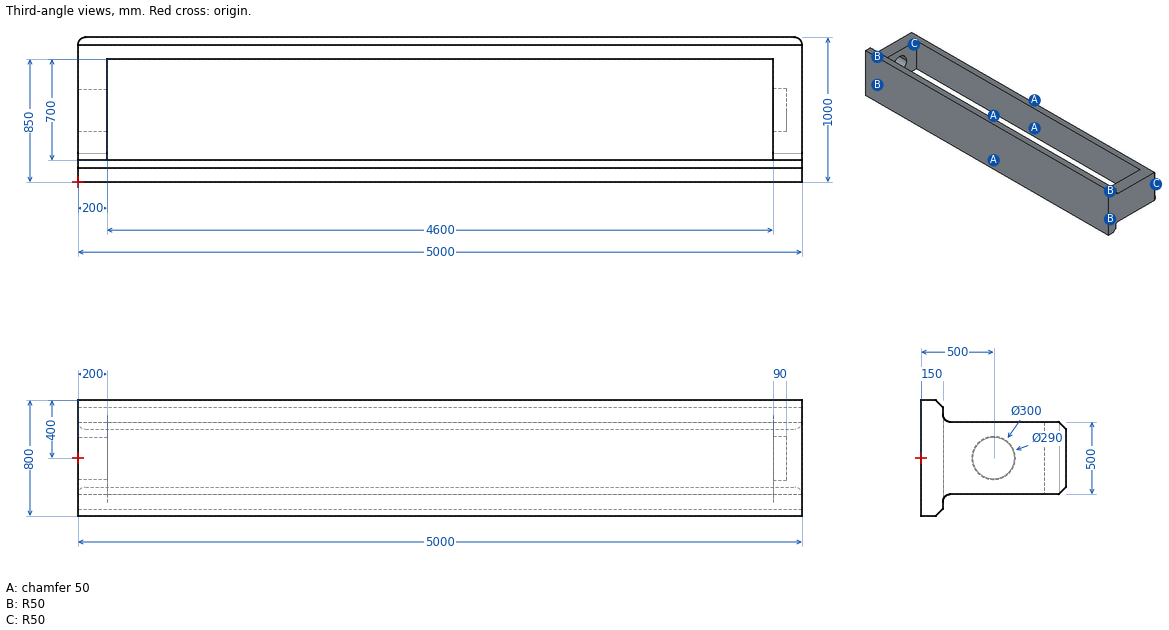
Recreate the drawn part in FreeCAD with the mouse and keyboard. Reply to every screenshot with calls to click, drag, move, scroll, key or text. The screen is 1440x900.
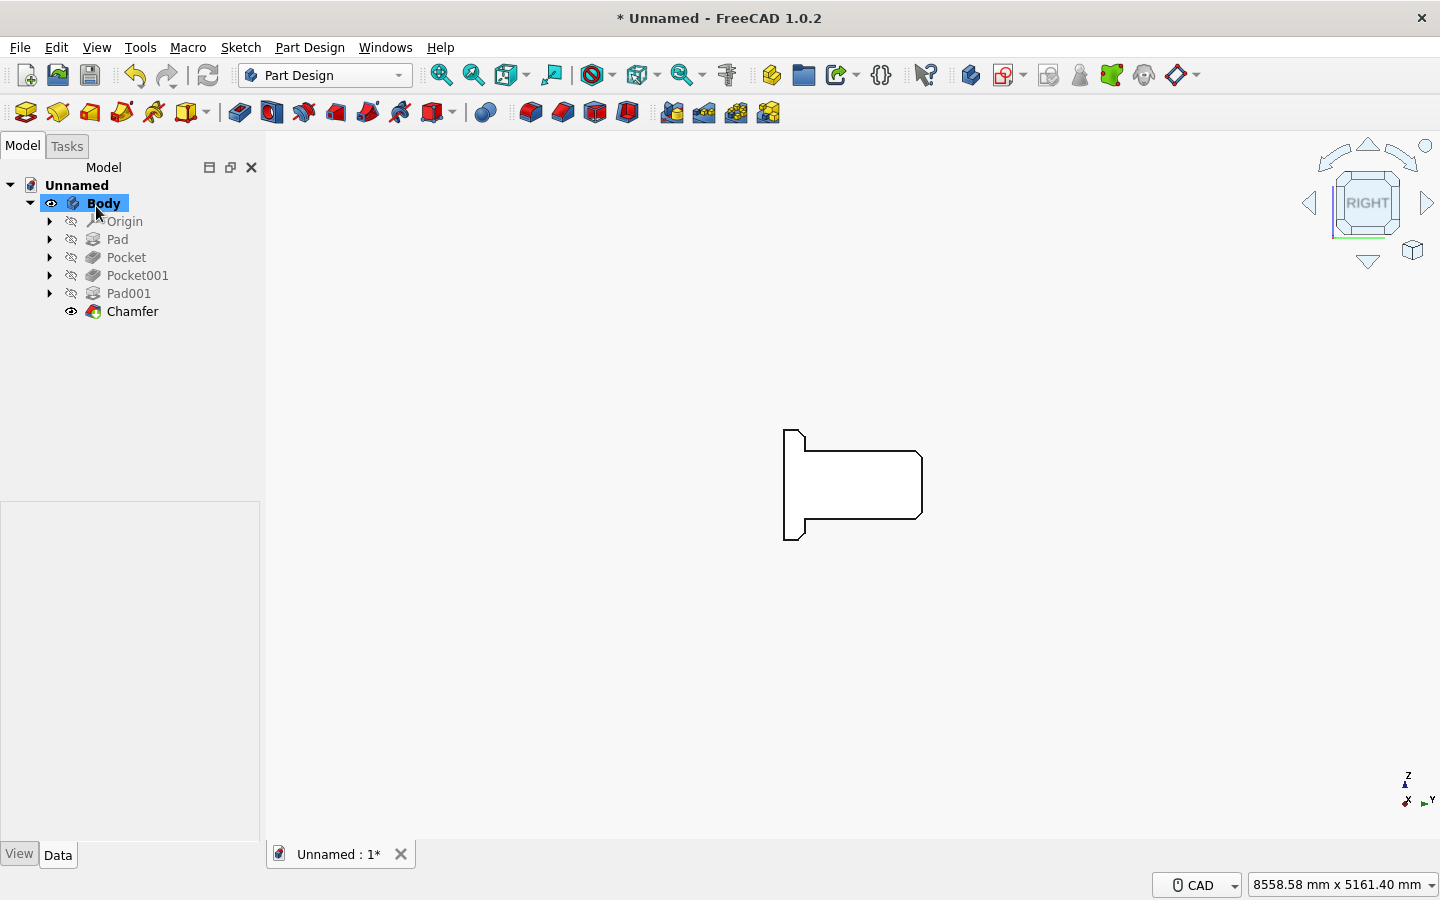
key(v)
key(f)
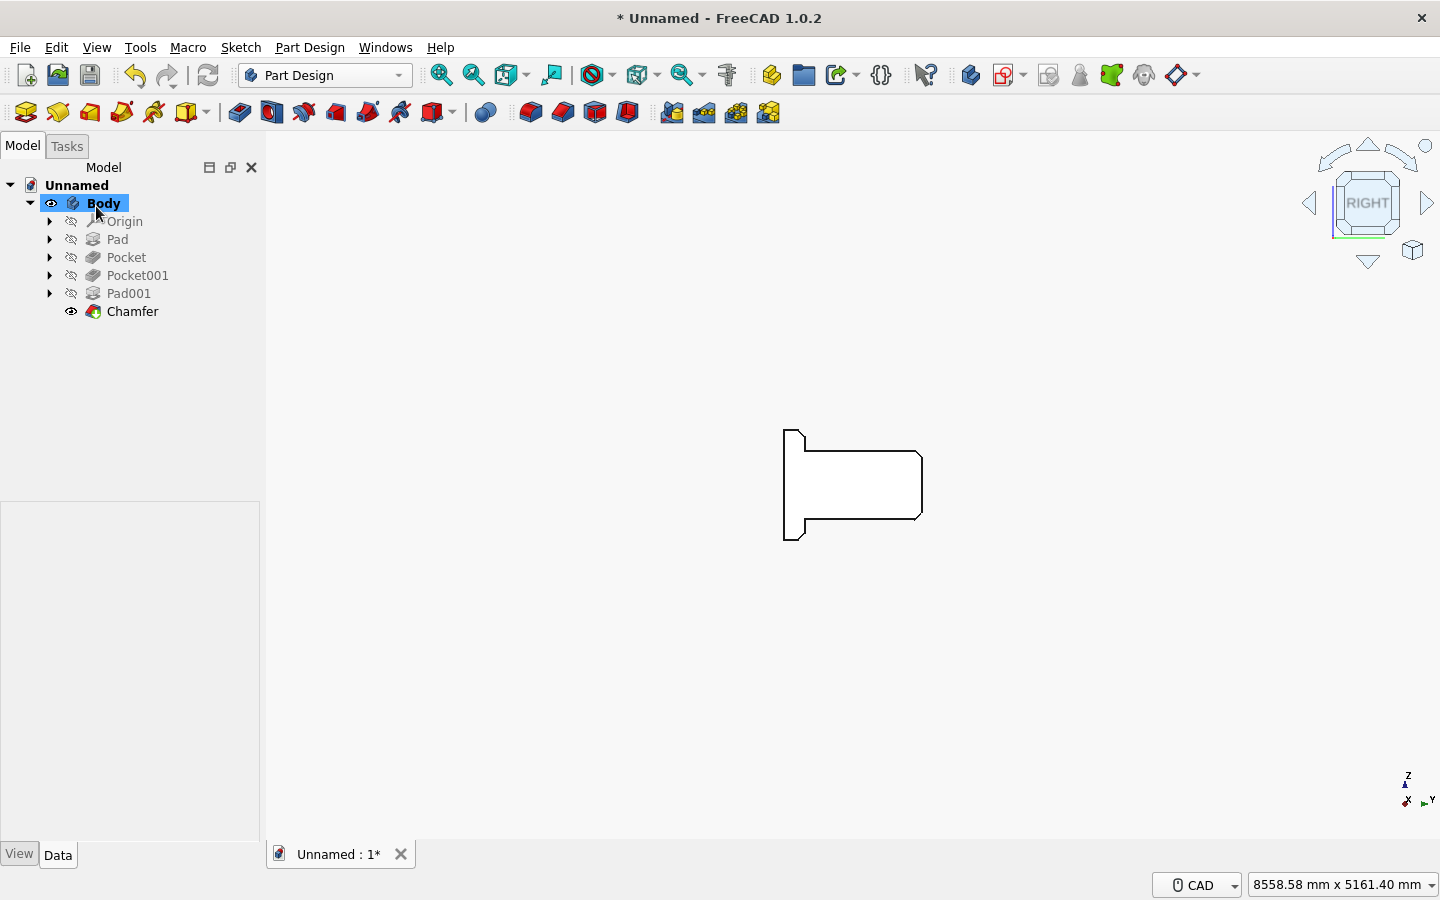
key(5)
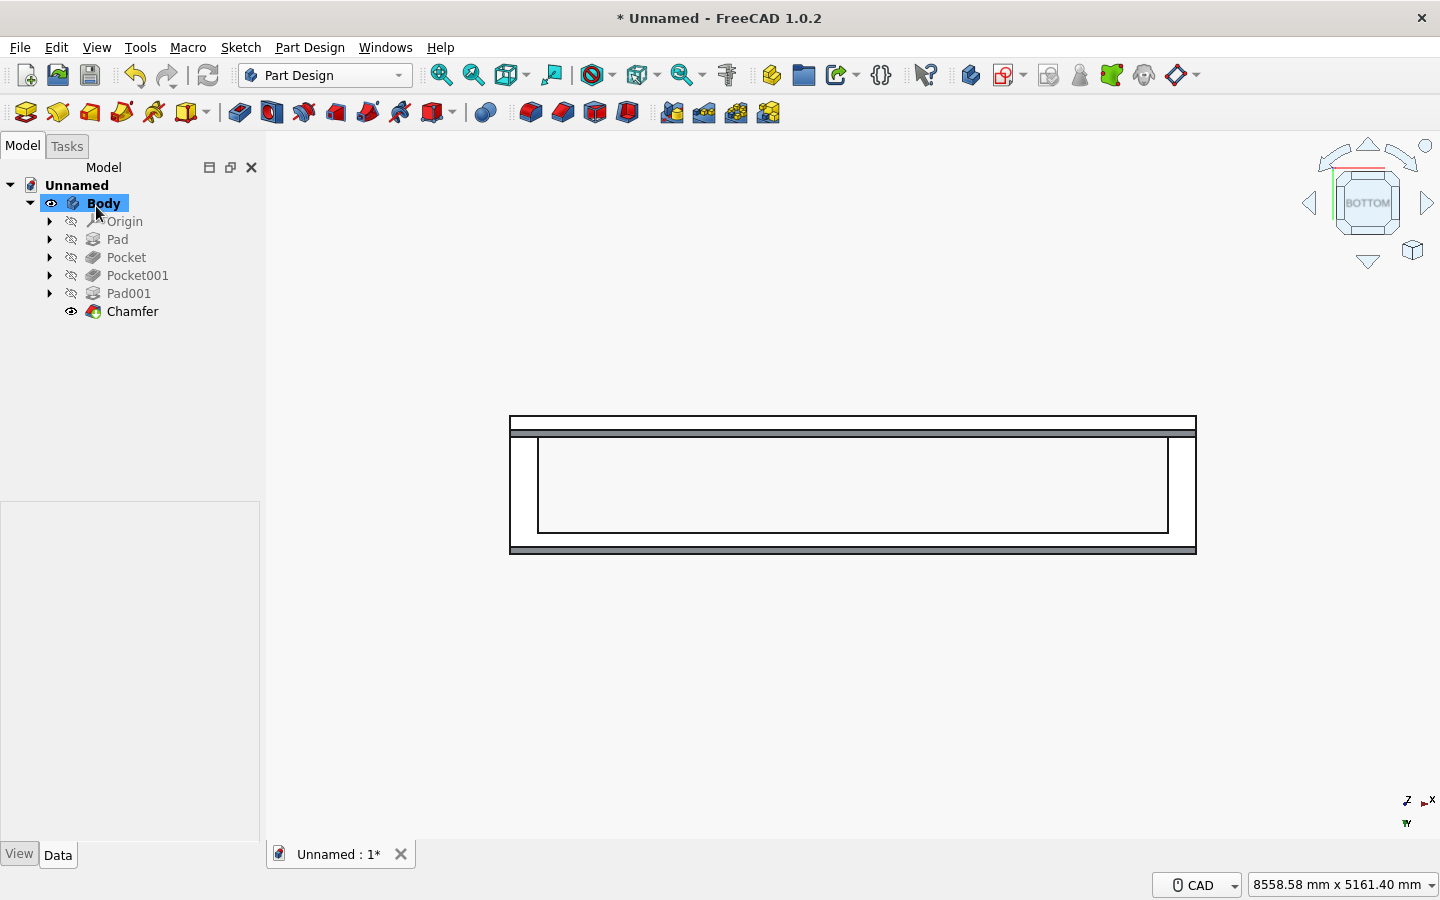
key(4)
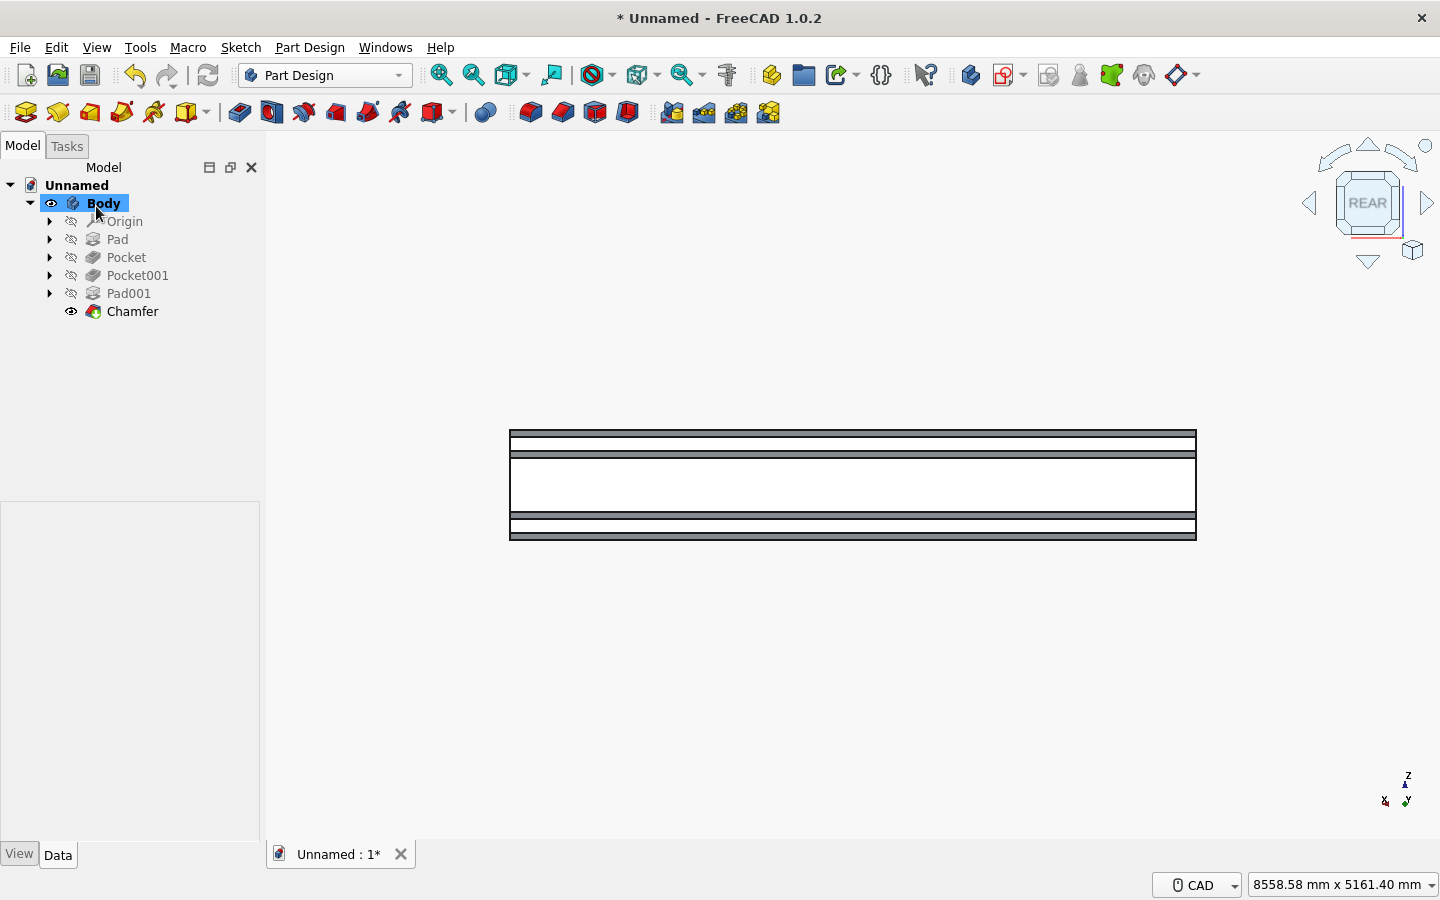
key(6)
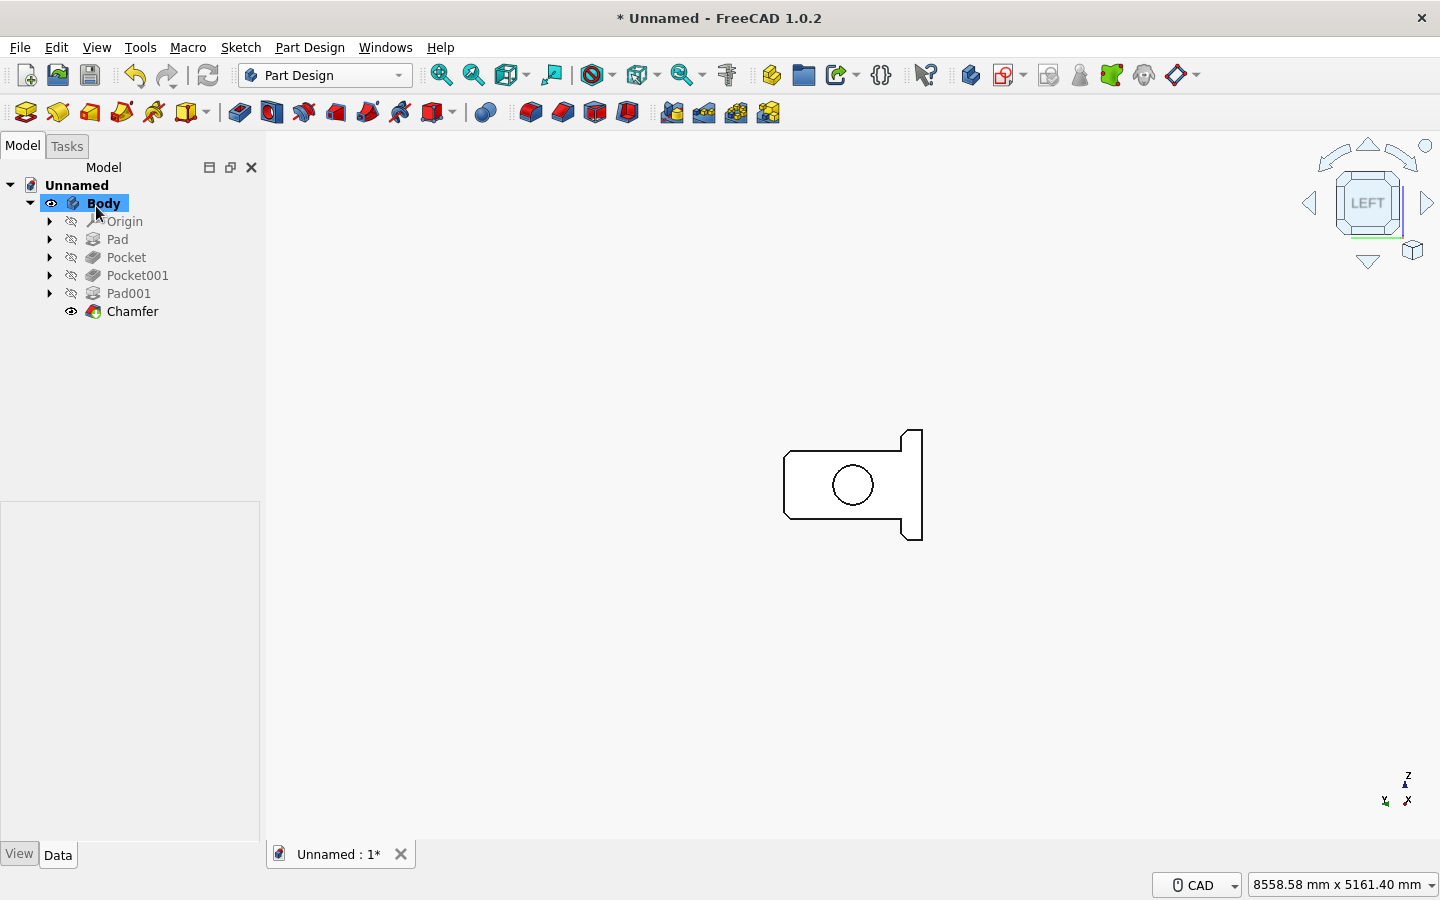
click(442, 76)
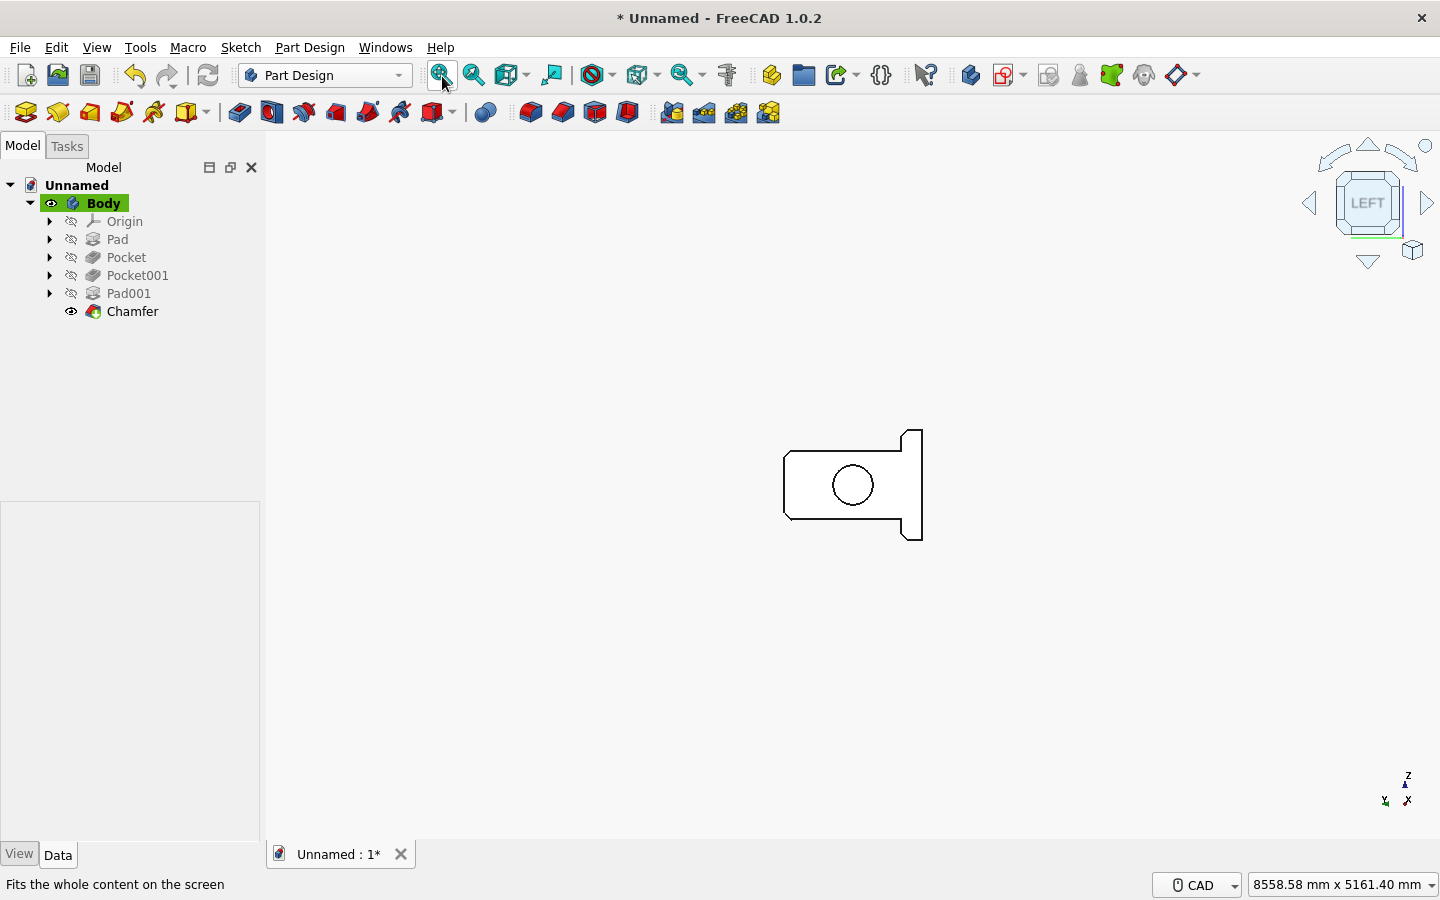
key(v)
key(3)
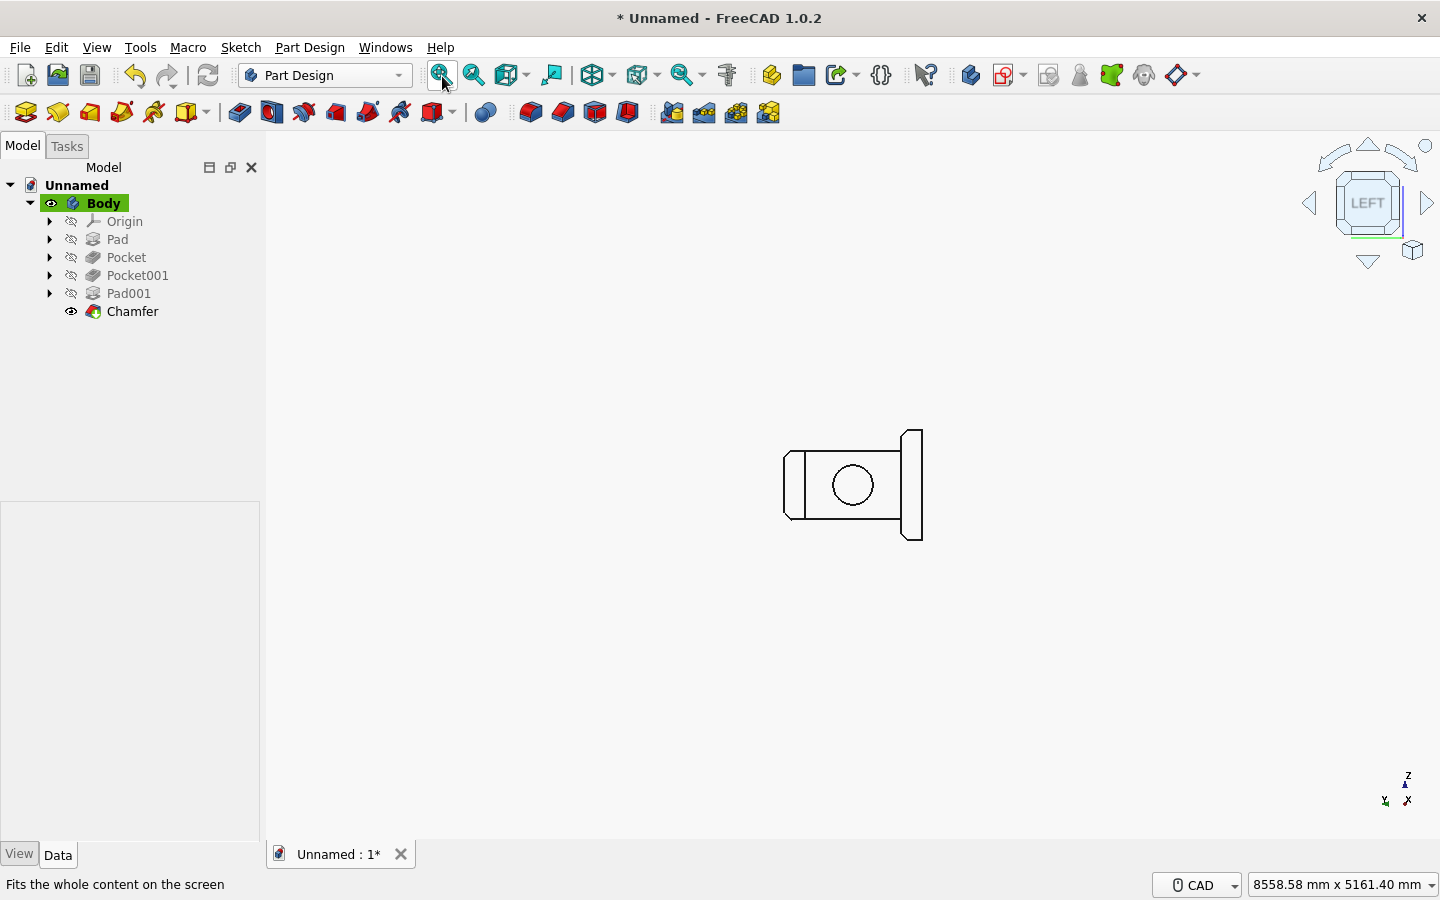
key(0)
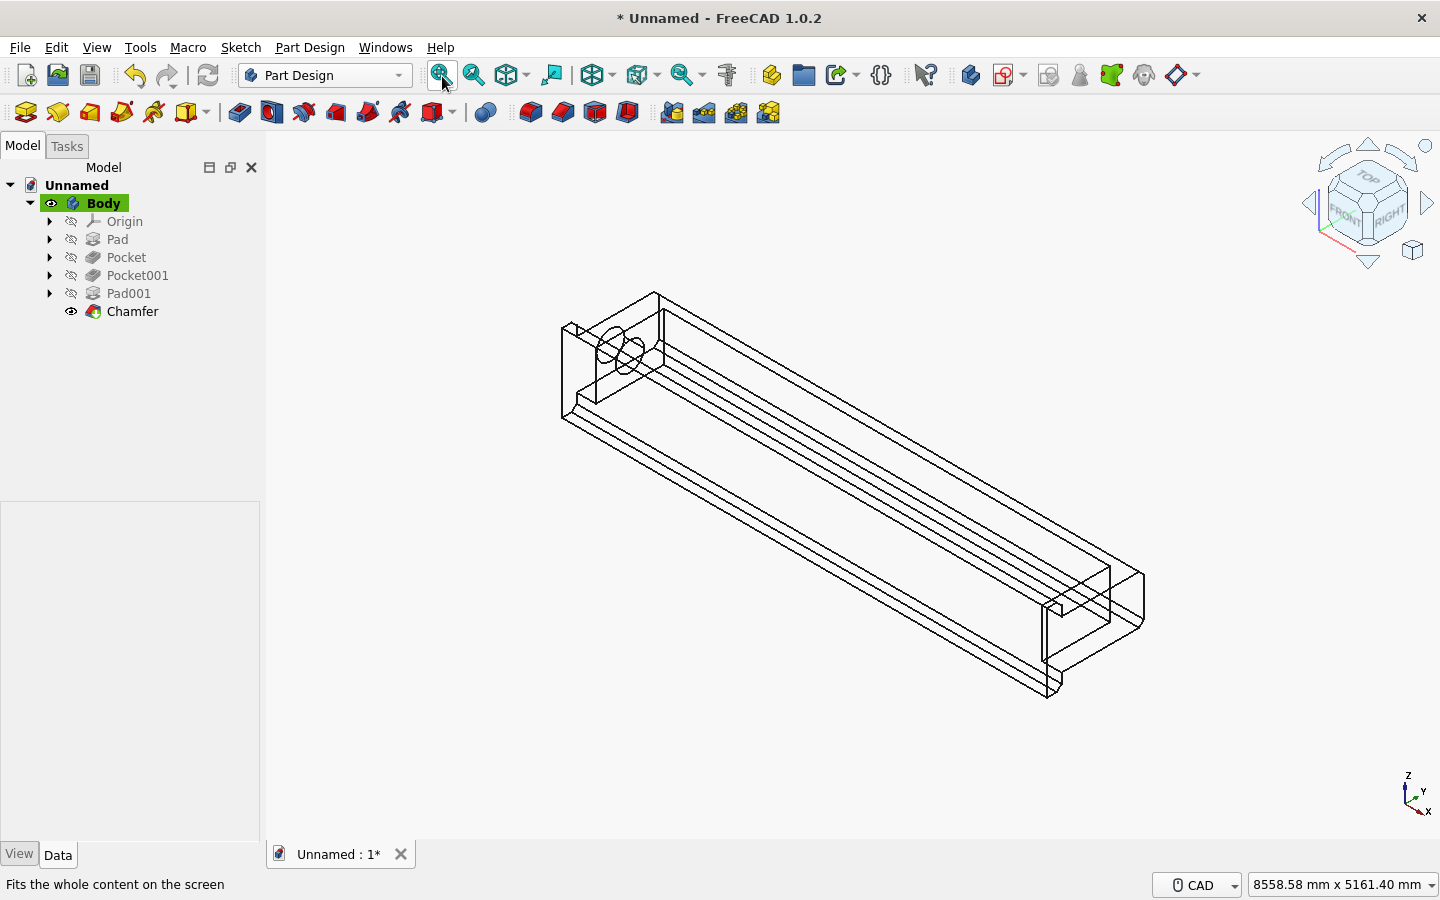
click(1054, 611)